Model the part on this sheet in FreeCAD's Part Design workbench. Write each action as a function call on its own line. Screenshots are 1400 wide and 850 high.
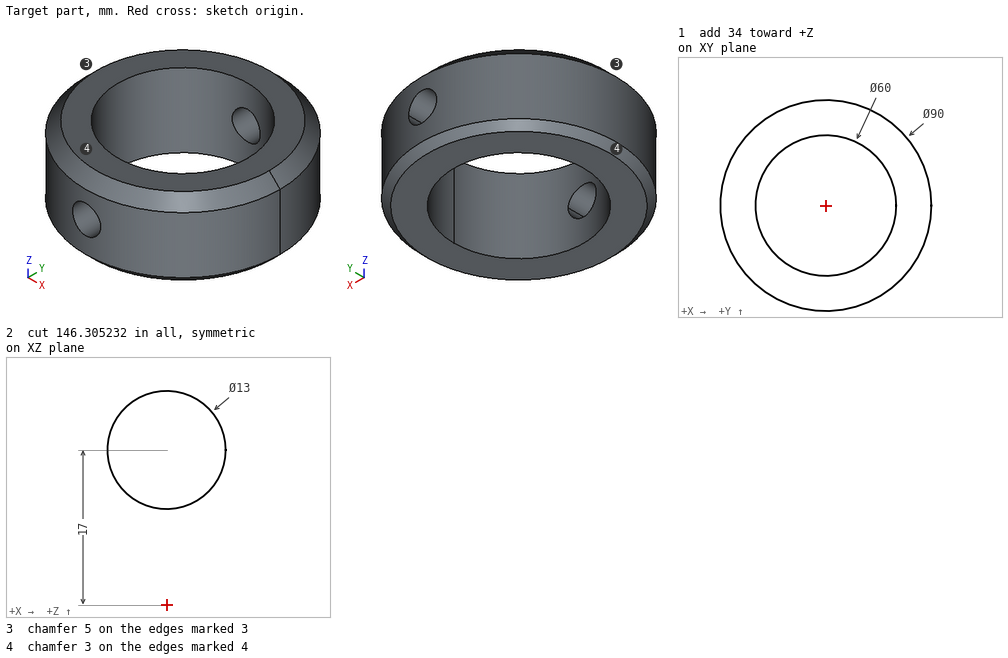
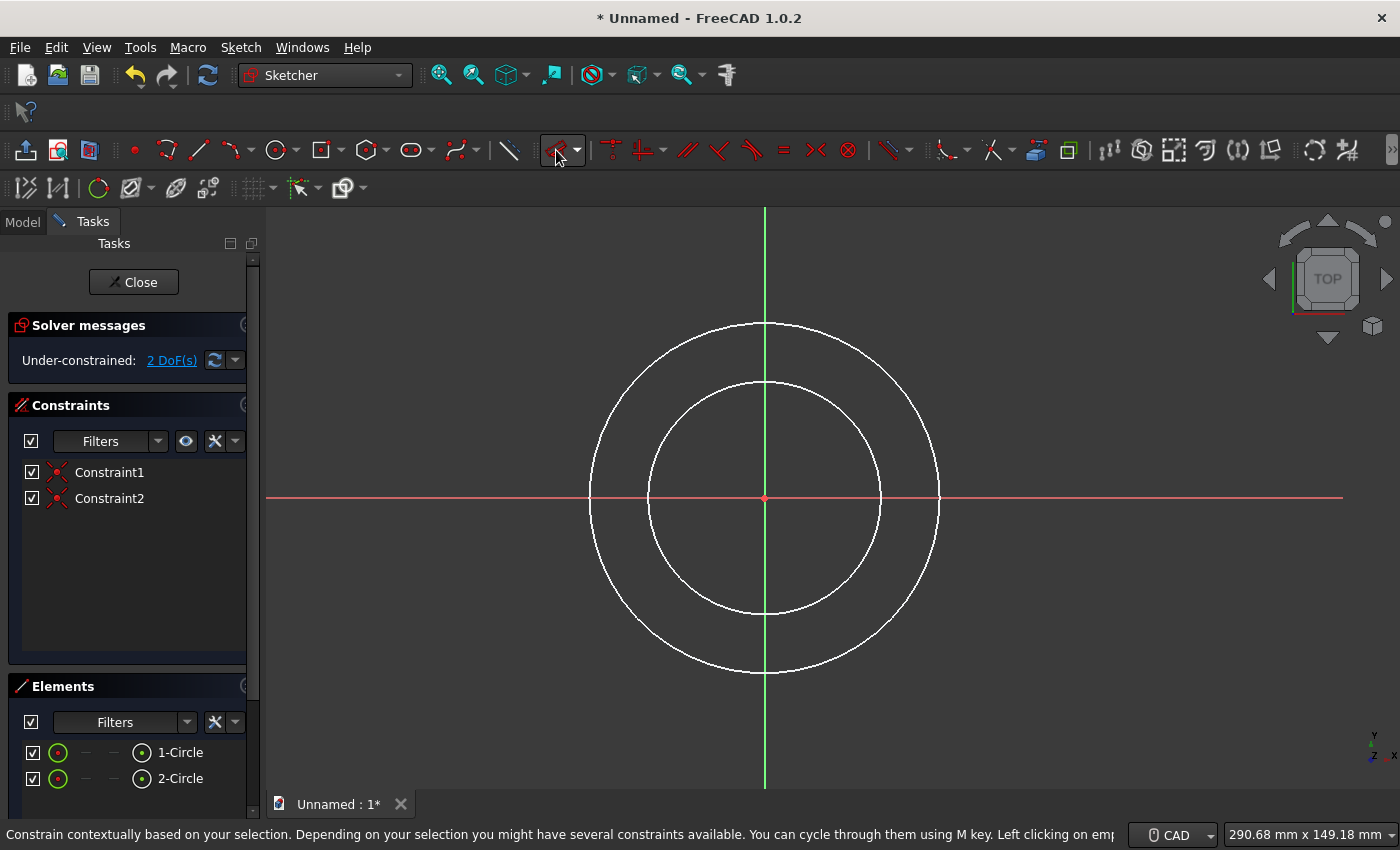
click(888, 374)
click(911, 351)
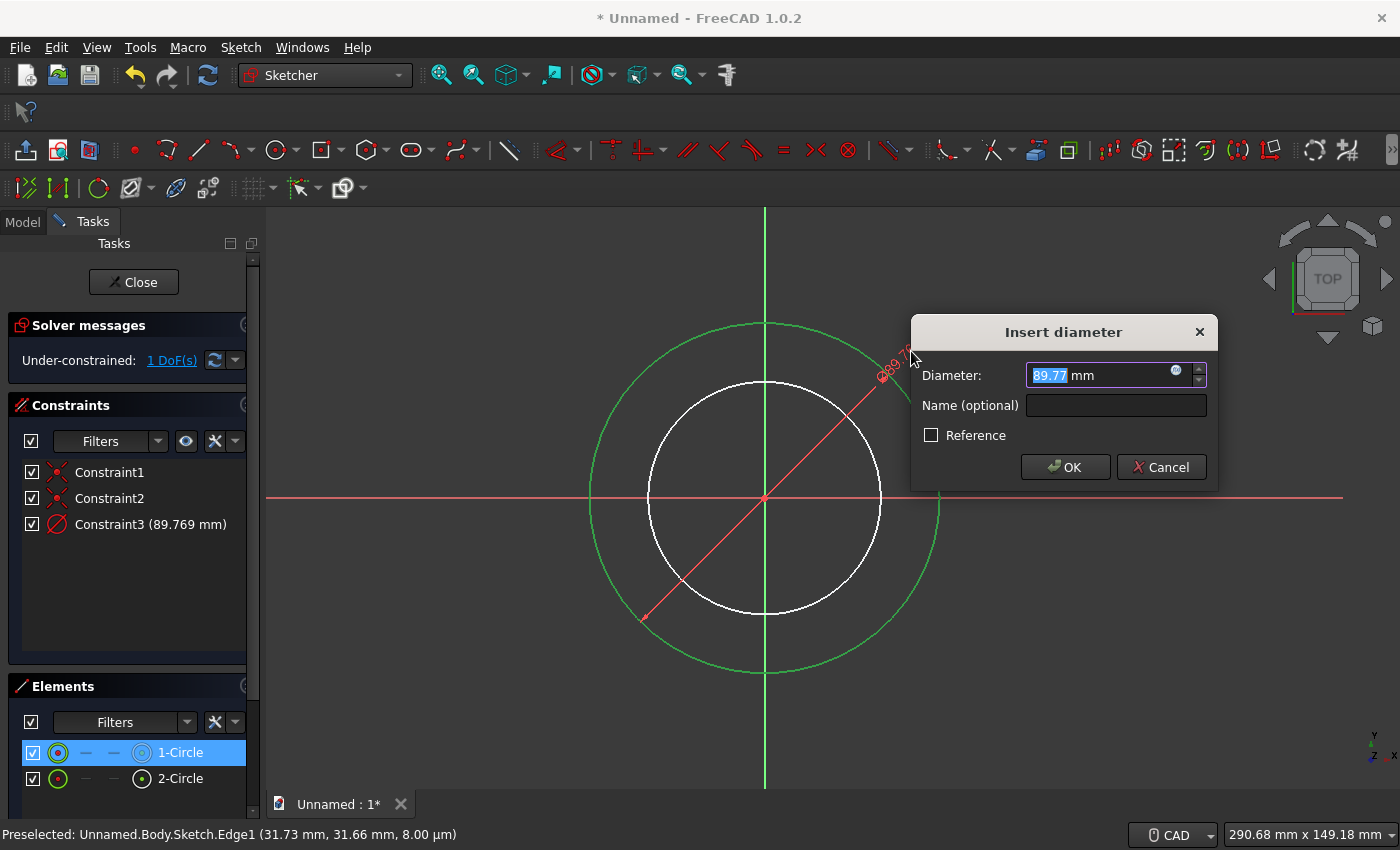
text(90)
key(Return)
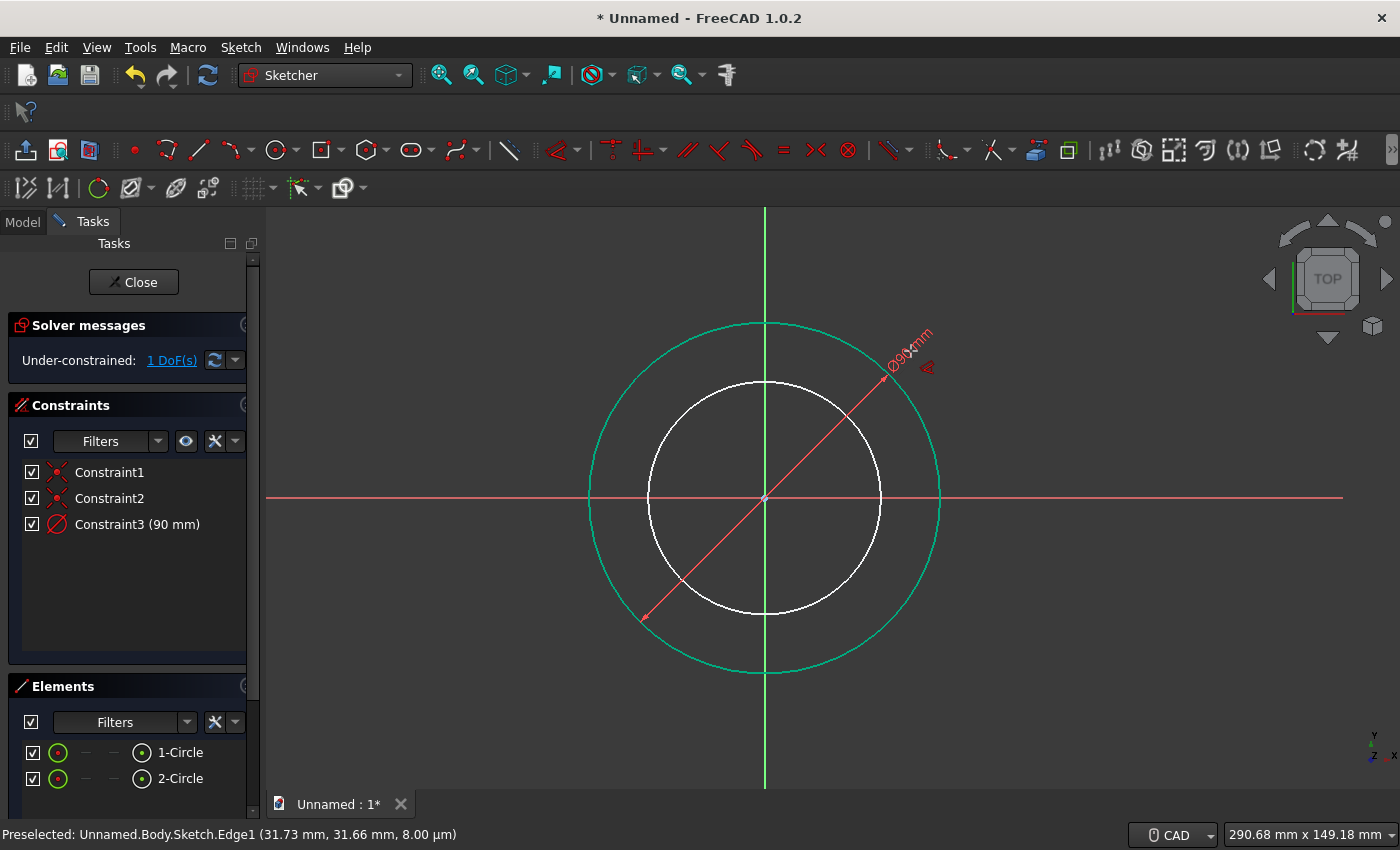
click(847, 416)
click(870, 393)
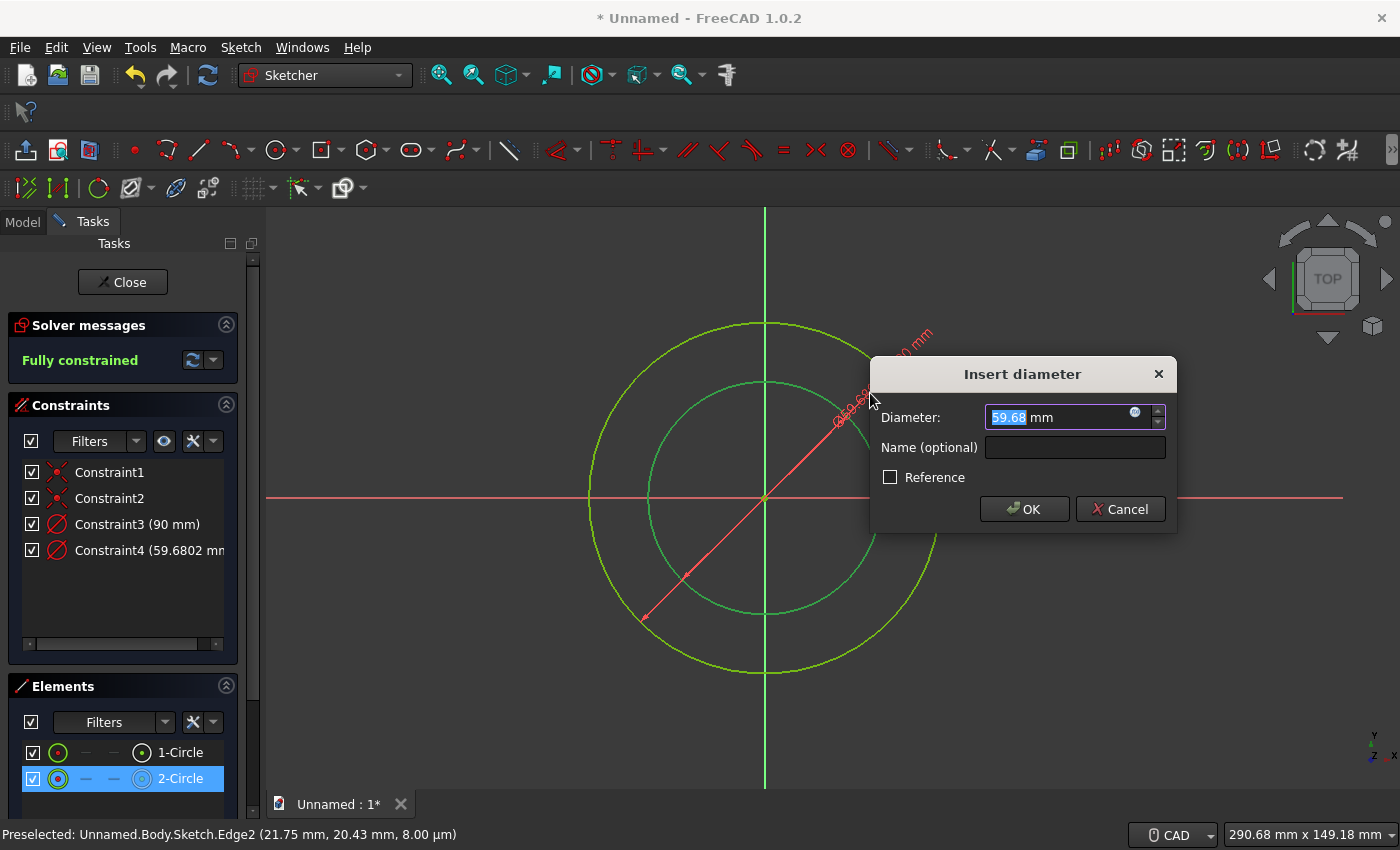
text(60)
key(Return)
key(Escape)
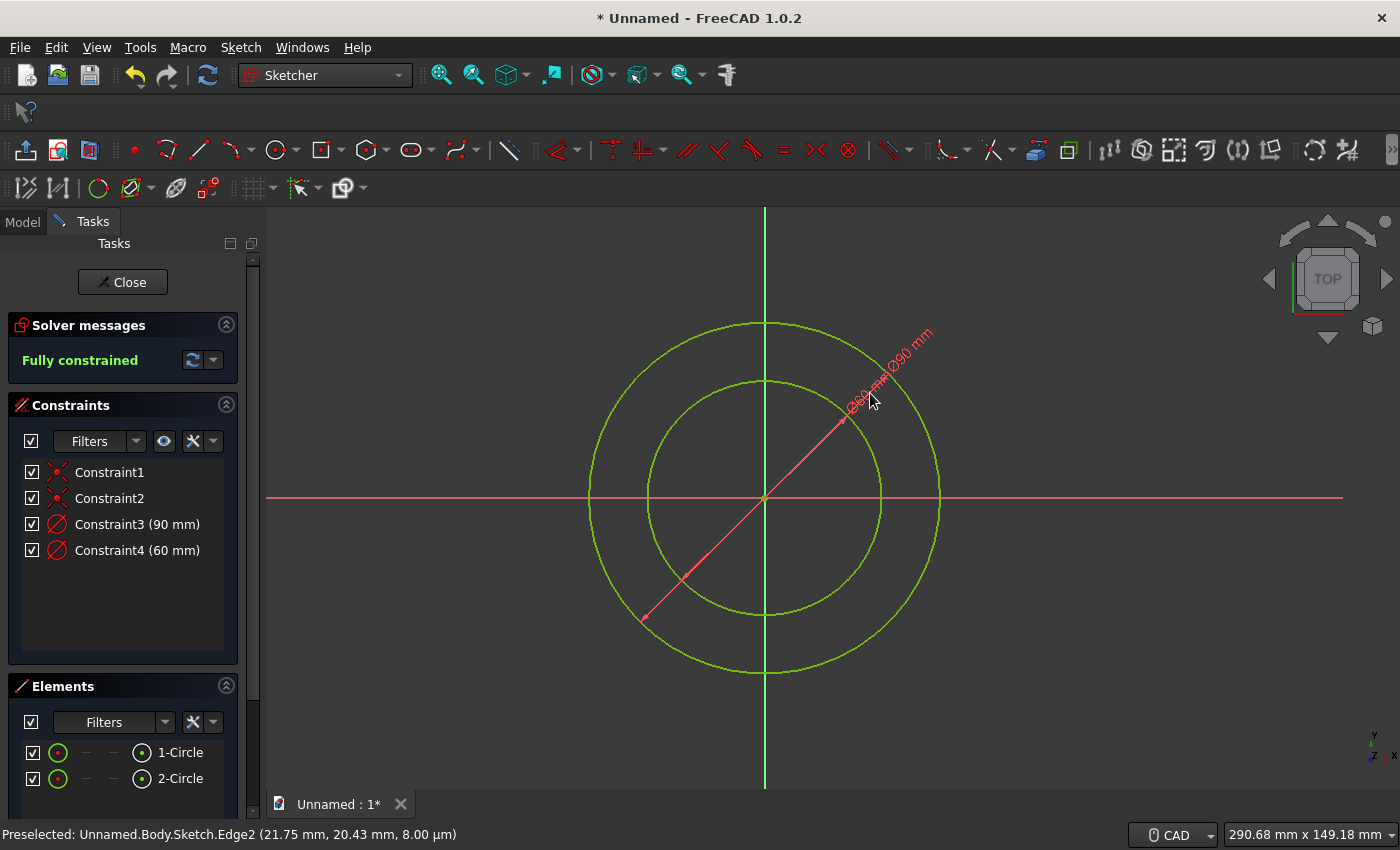
click(123, 282)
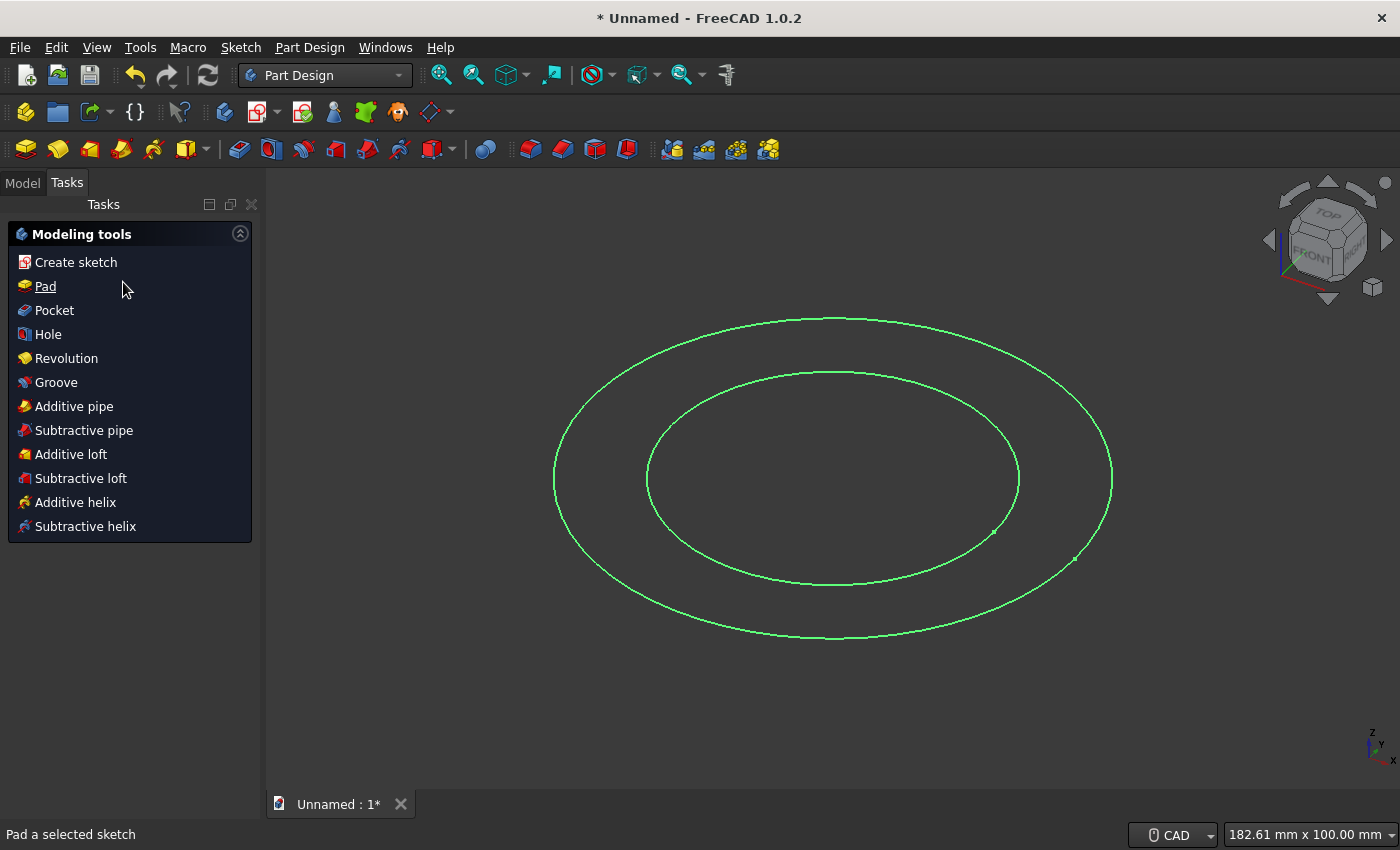
click(26, 150)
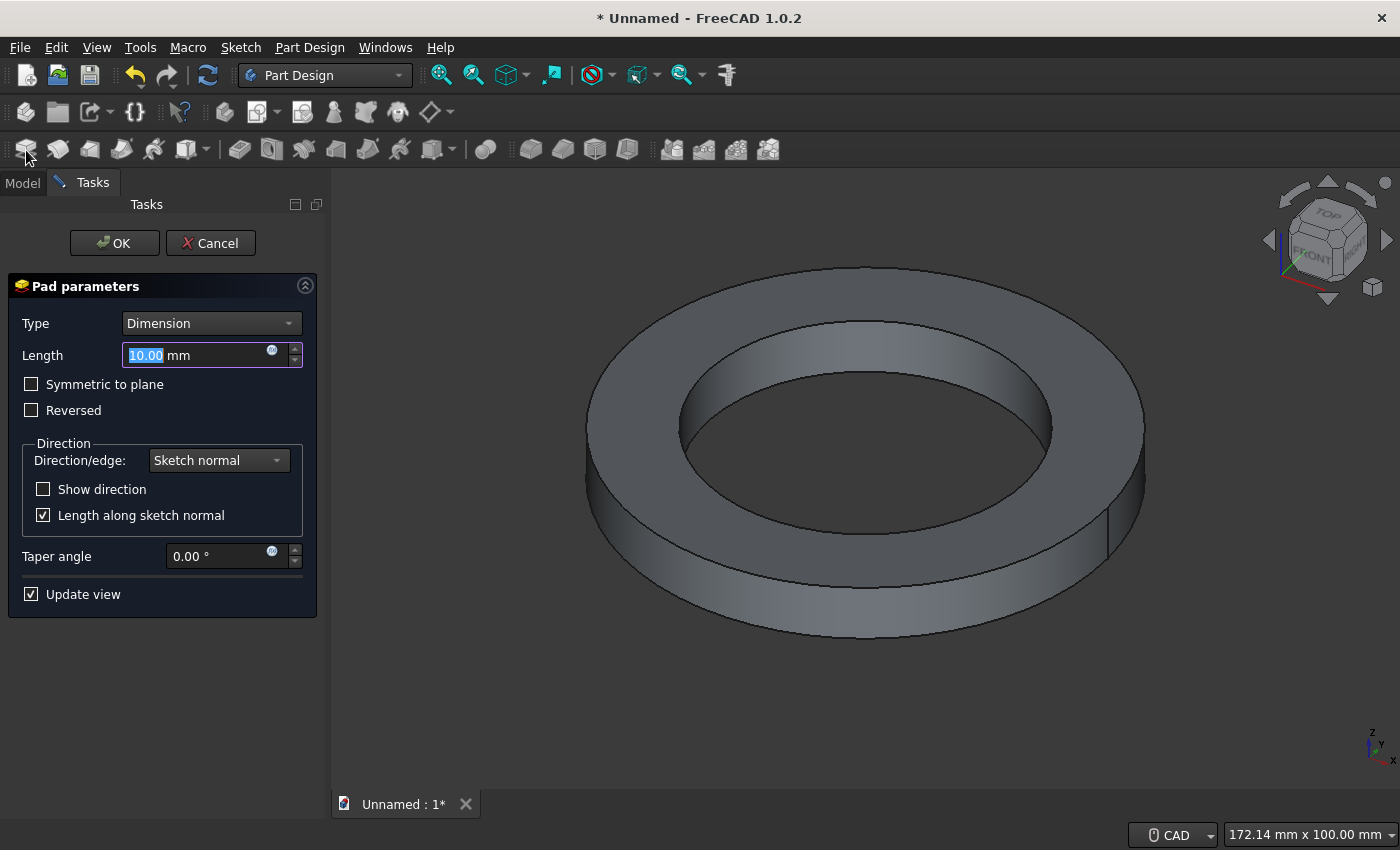
text(34)
key(Tab)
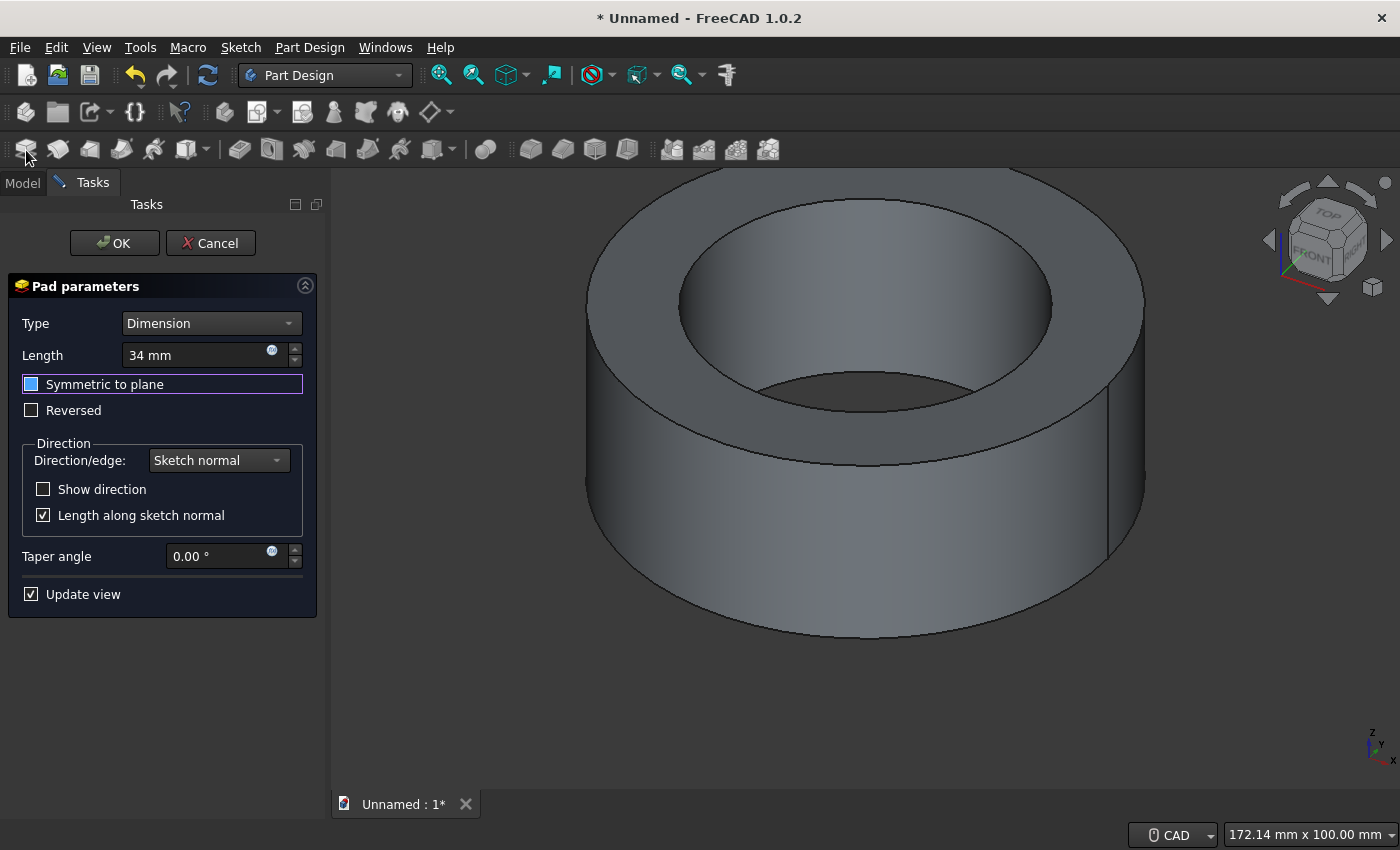
click(115, 243)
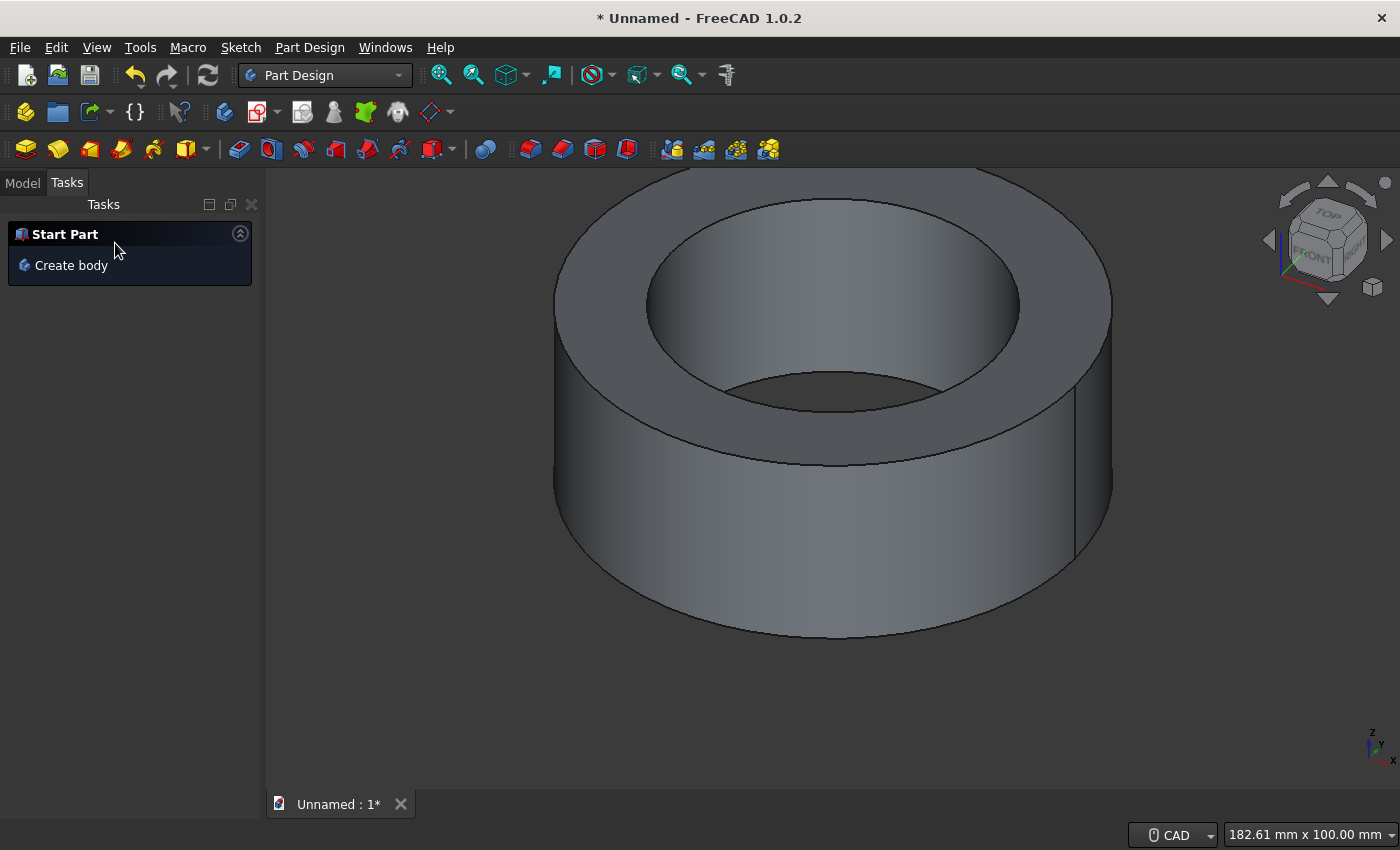
key(v)
key(f)